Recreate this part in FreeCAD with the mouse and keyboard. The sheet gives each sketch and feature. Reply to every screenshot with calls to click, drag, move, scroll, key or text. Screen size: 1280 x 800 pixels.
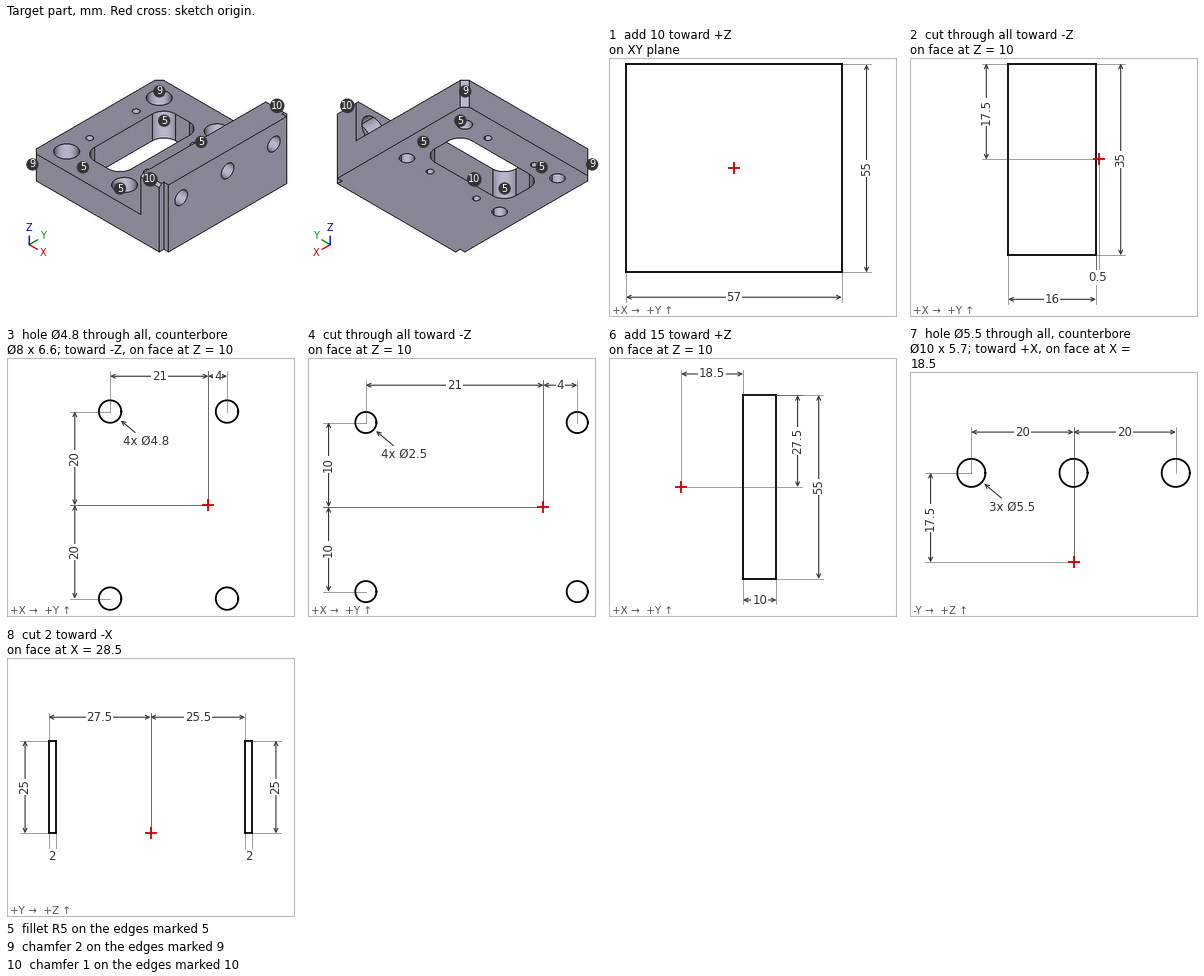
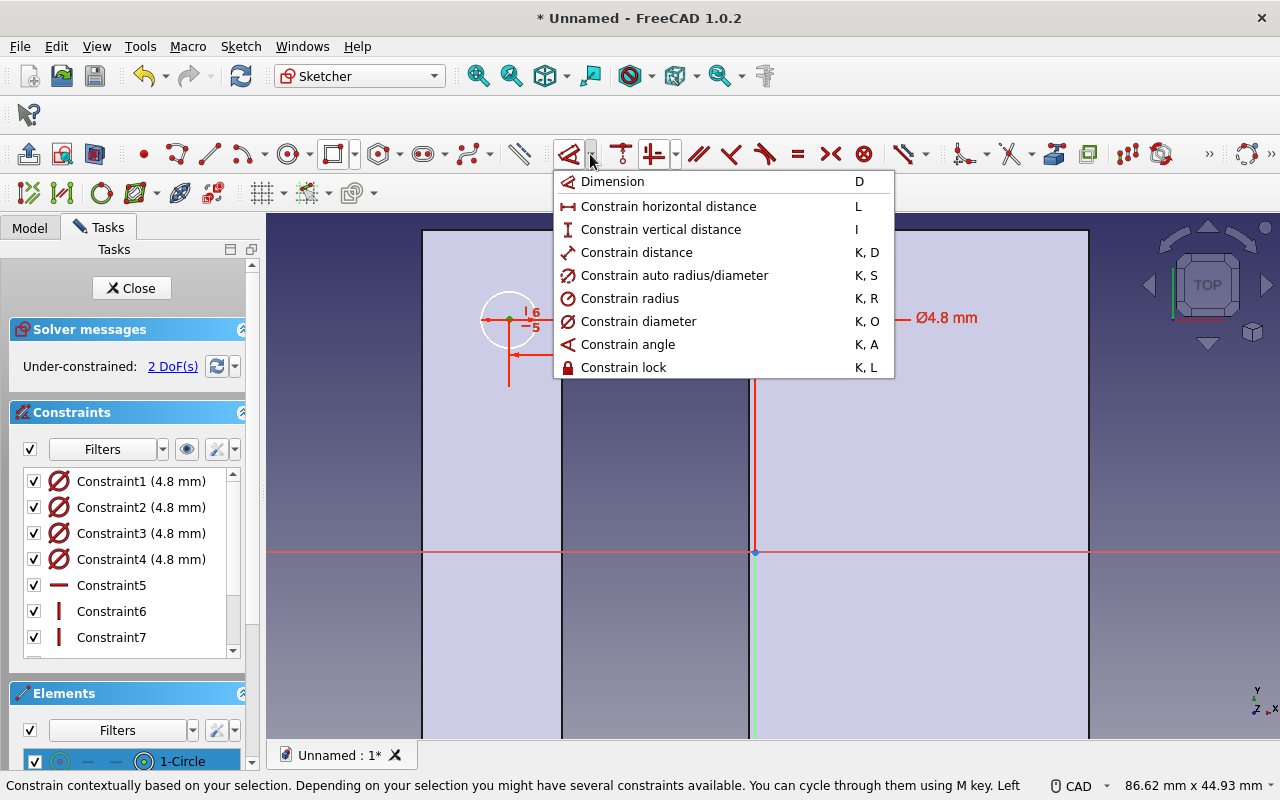
click(724, 230)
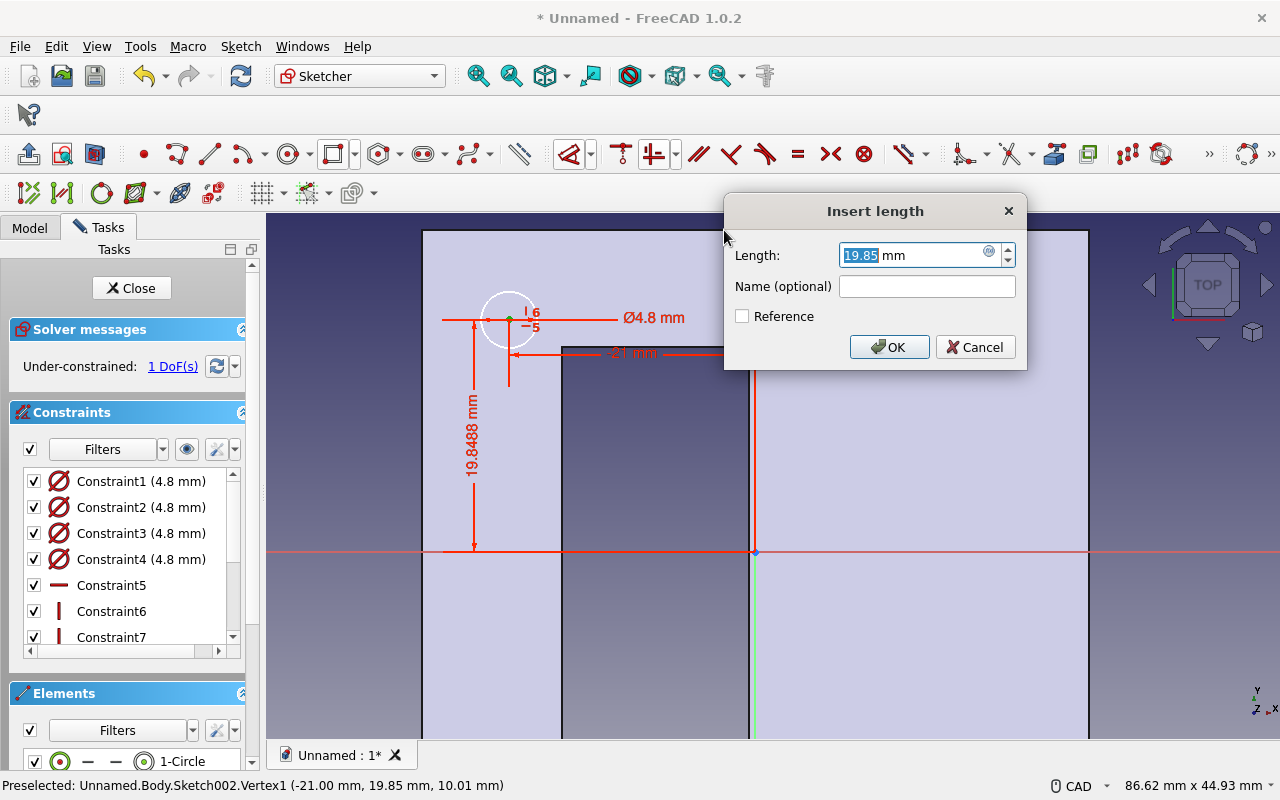
text(20)
key(Return)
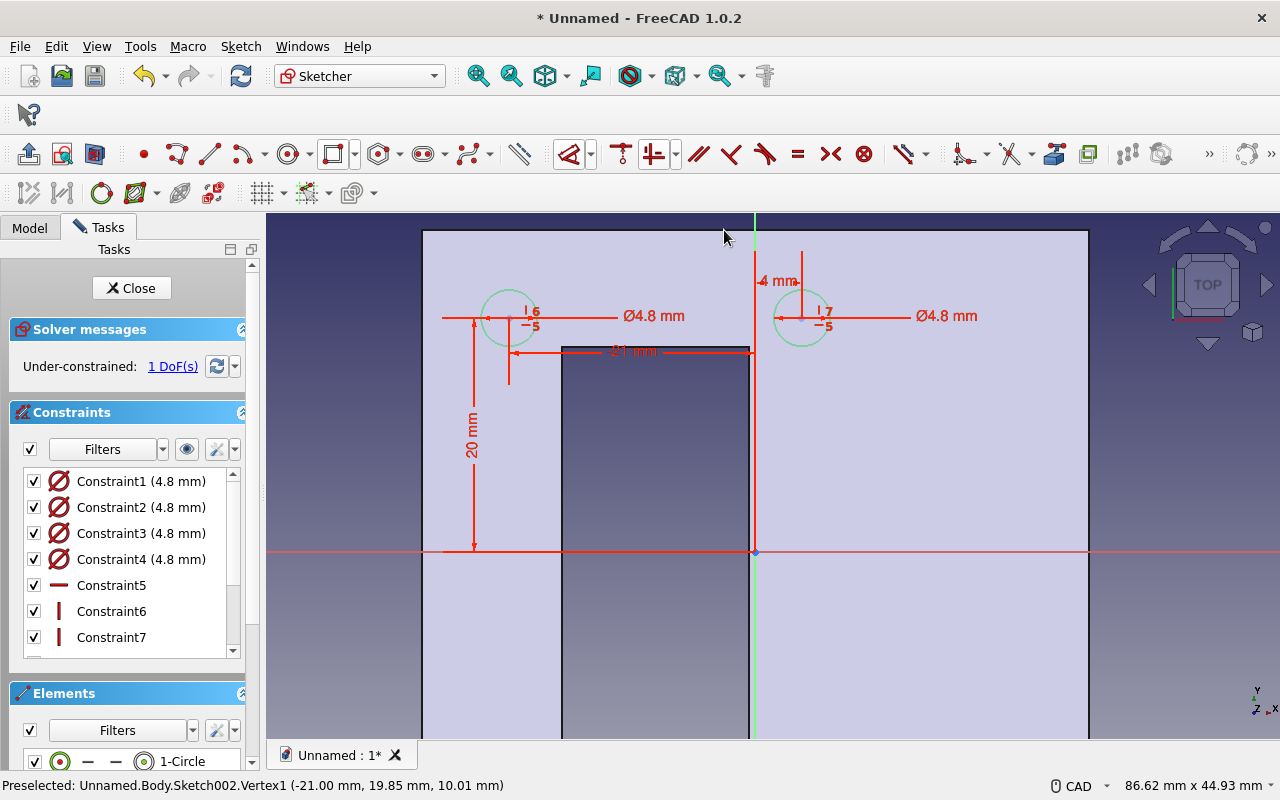
scroll(804, 321, down, 2)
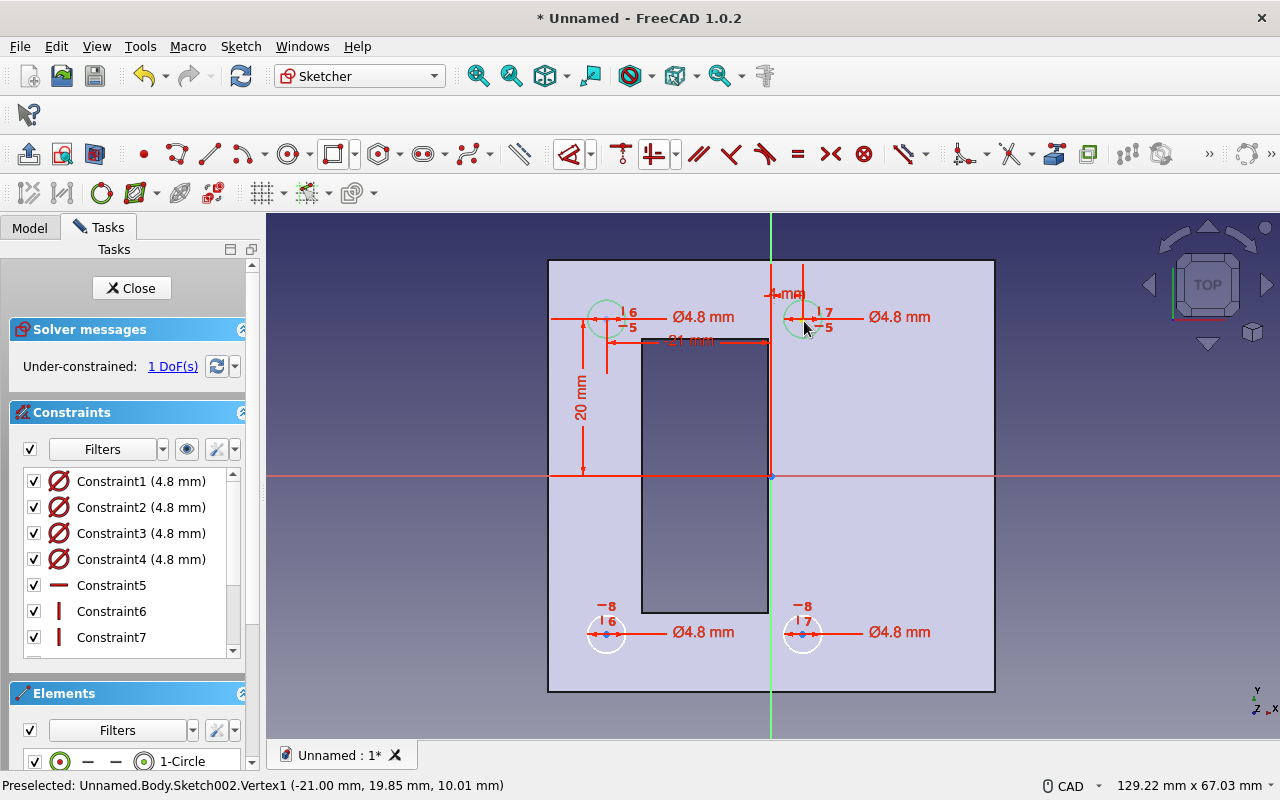
click(607, 634)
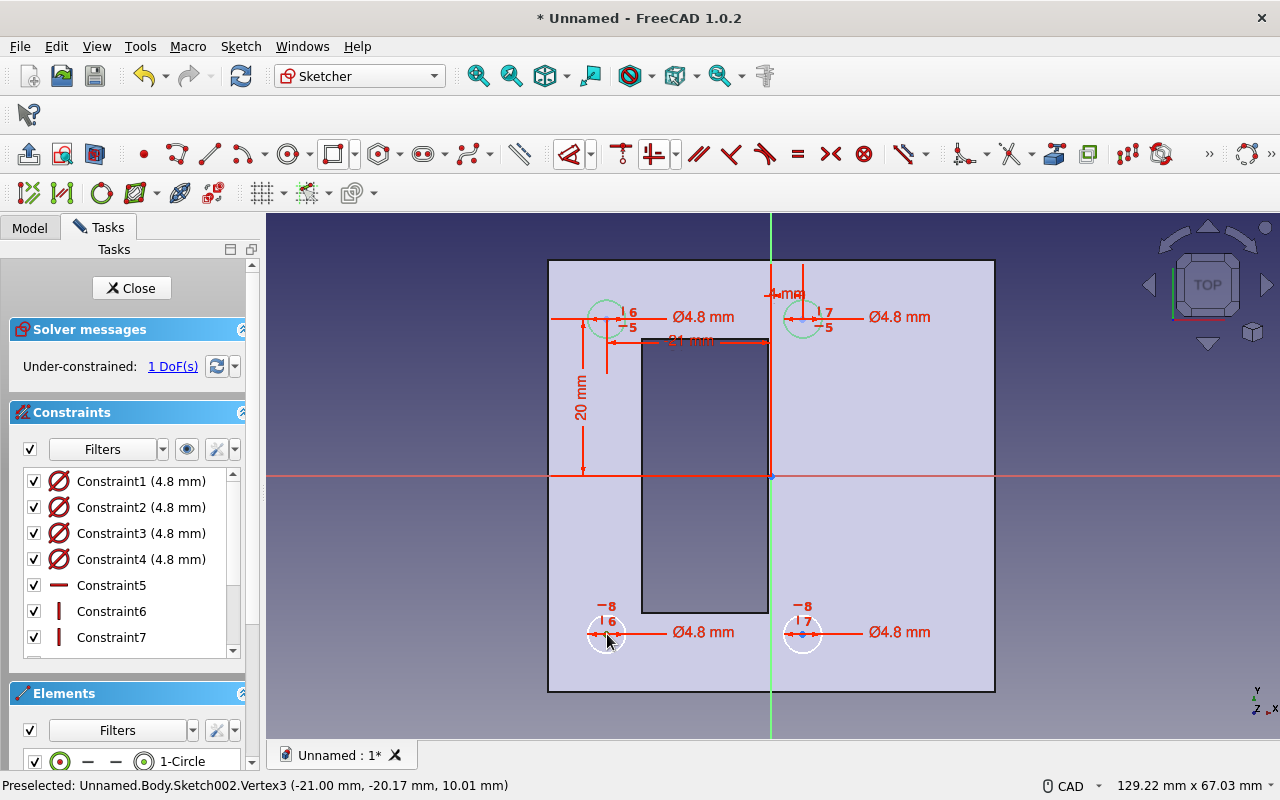
key(i)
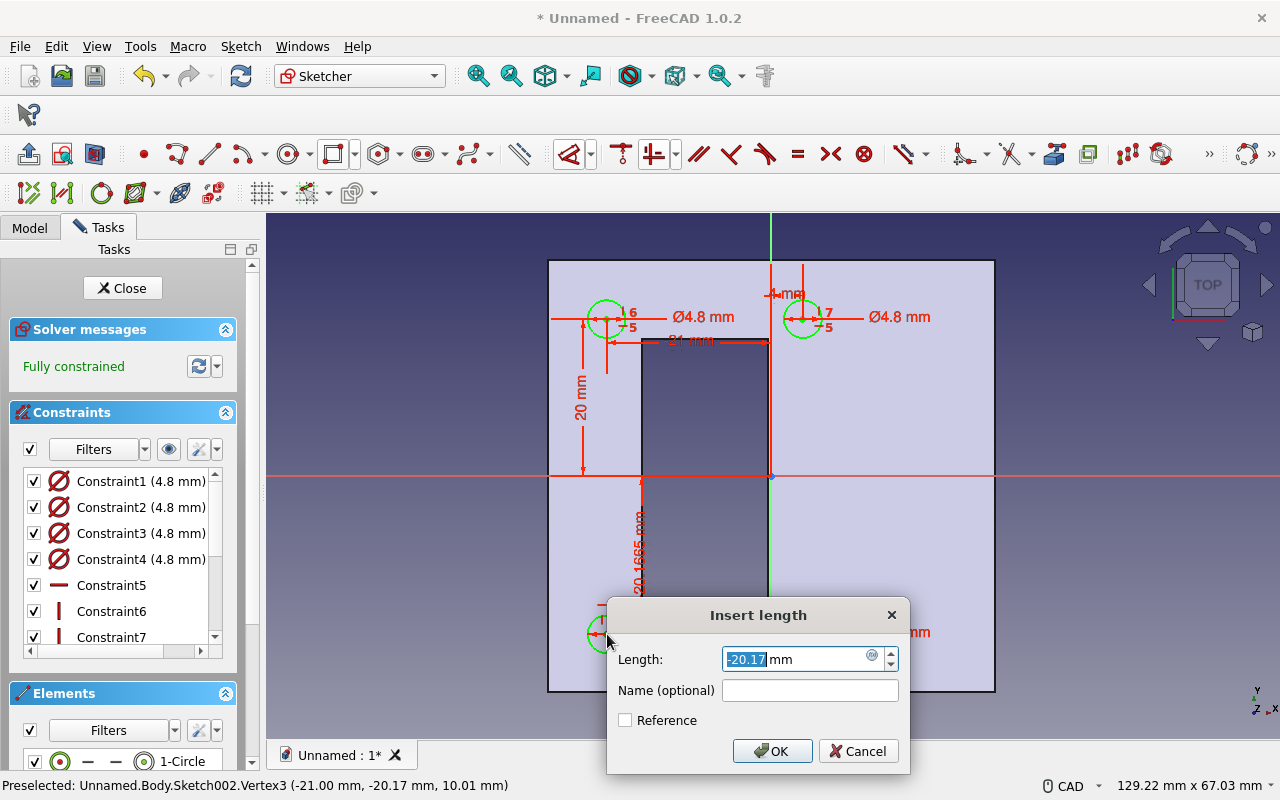
text(-20)
key(Return)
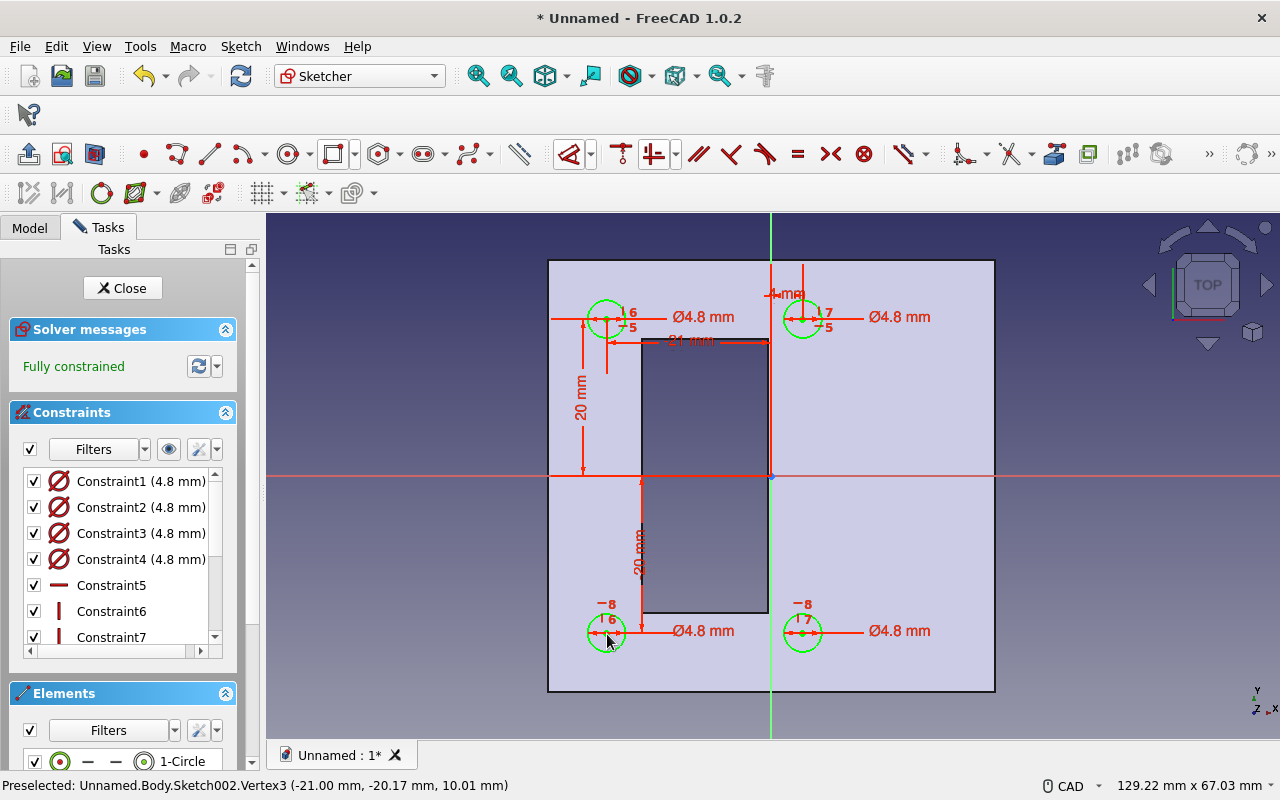
click(123, 288)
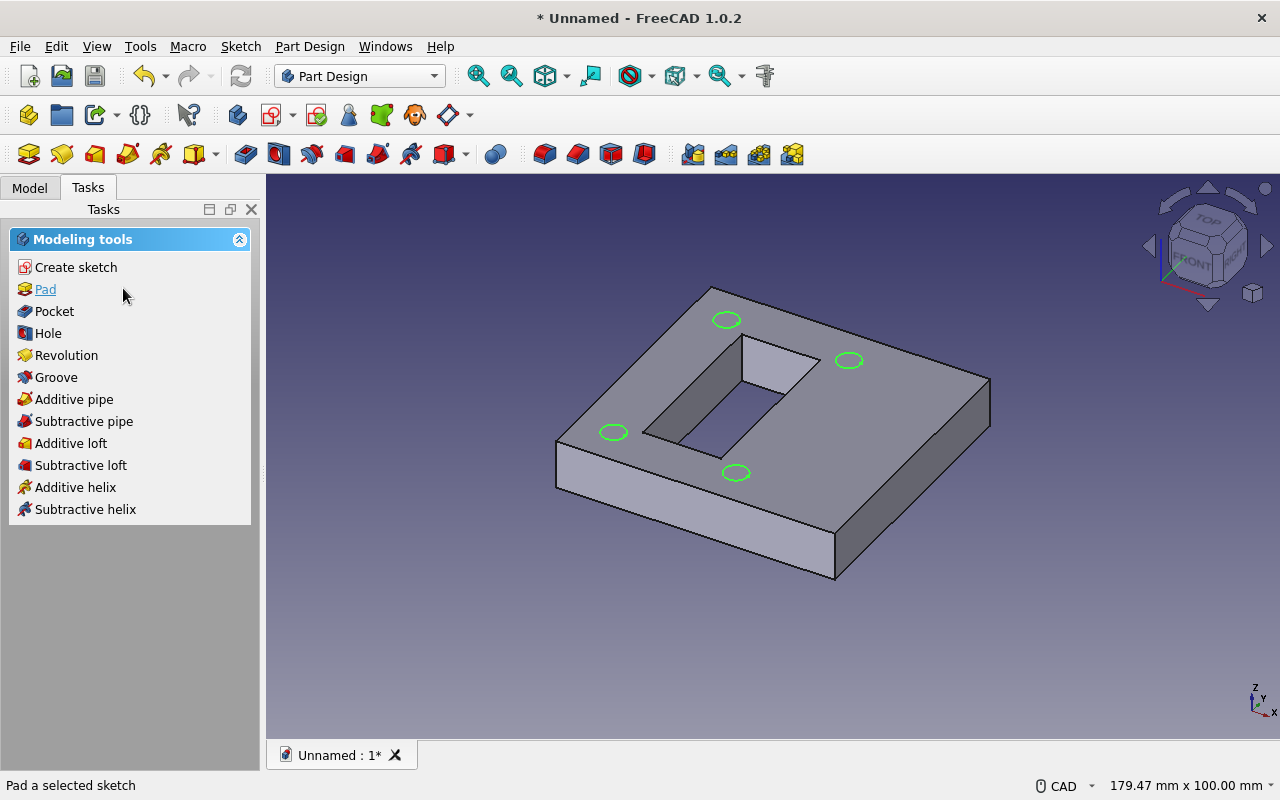
click(279, 154)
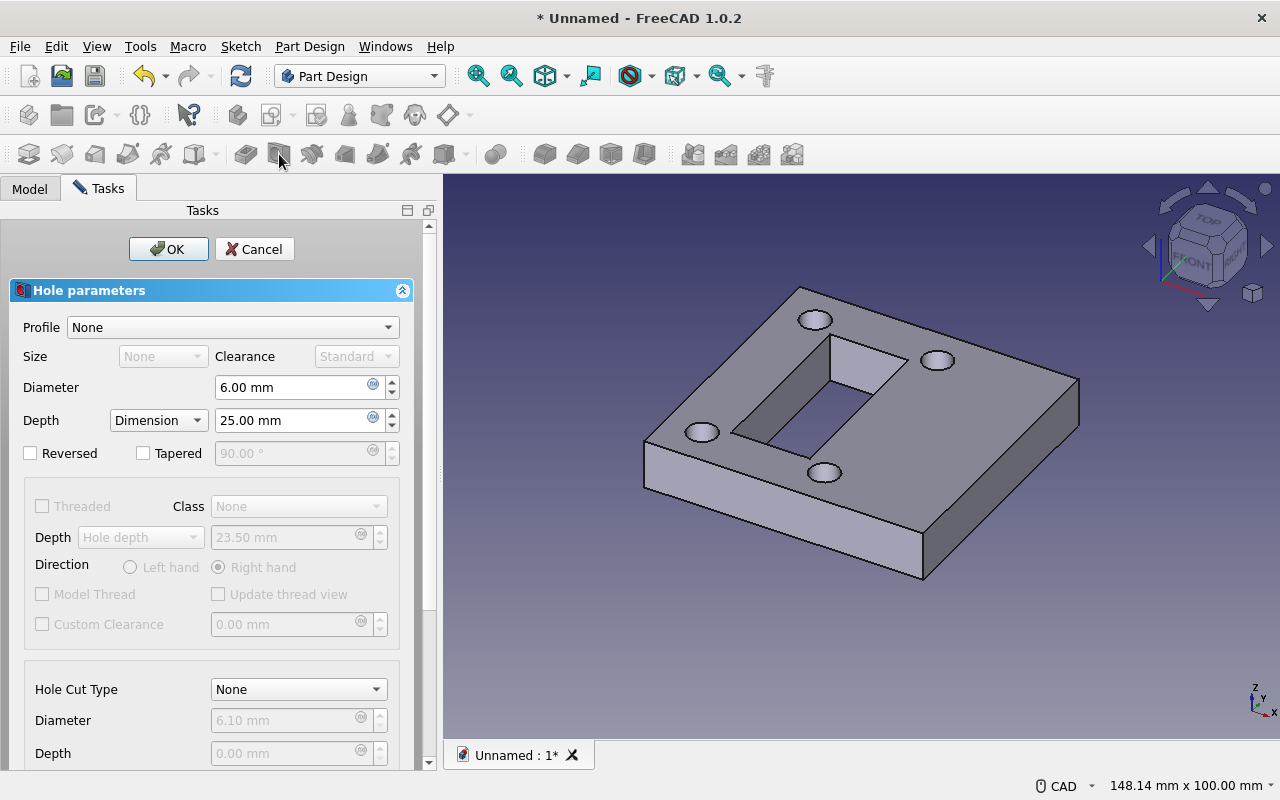
triple_click(300, 388)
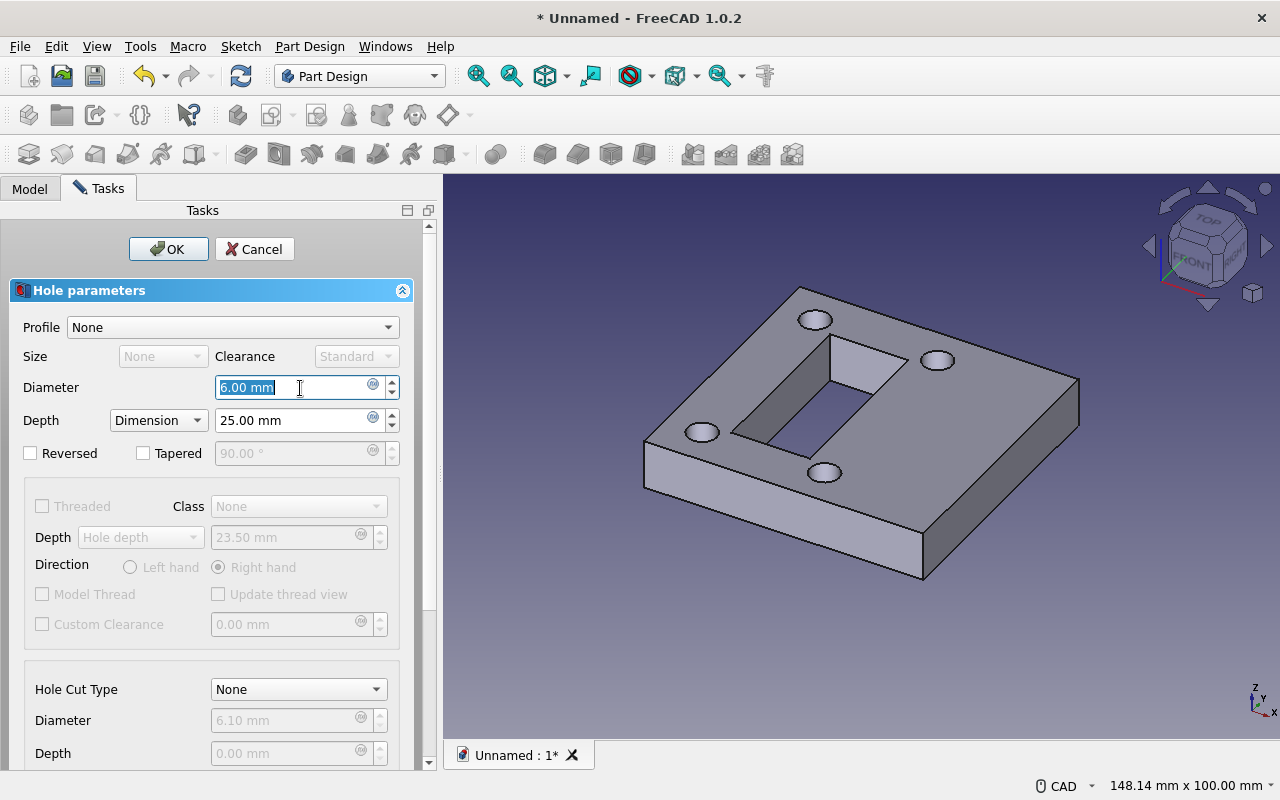
text(4.8)
key(Tab)